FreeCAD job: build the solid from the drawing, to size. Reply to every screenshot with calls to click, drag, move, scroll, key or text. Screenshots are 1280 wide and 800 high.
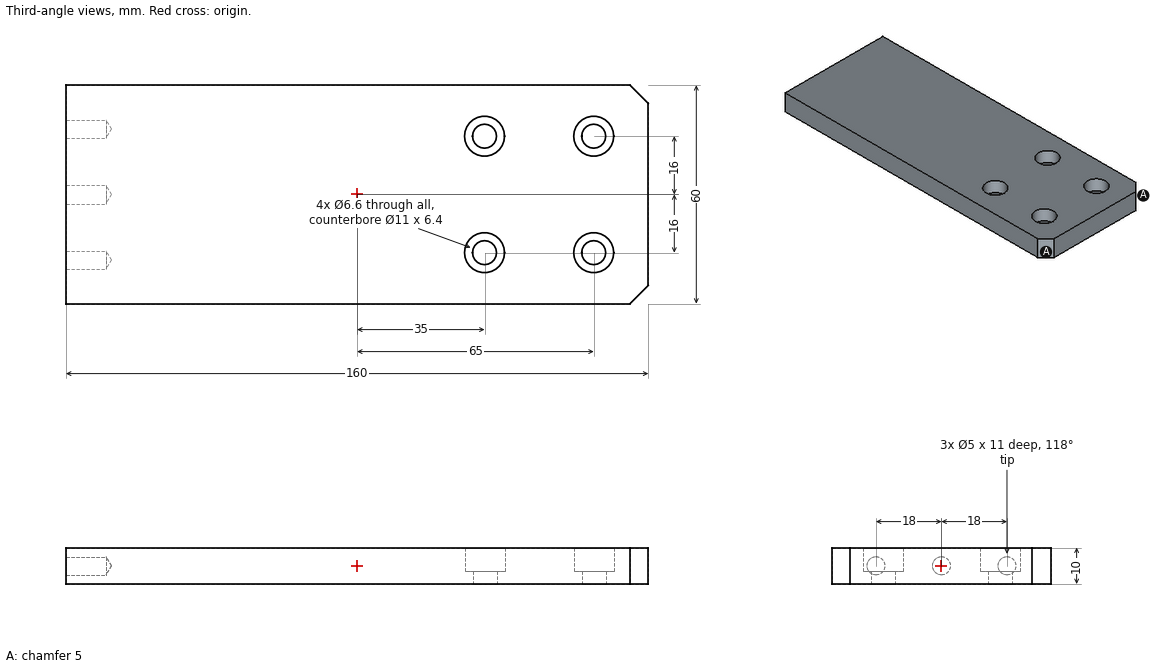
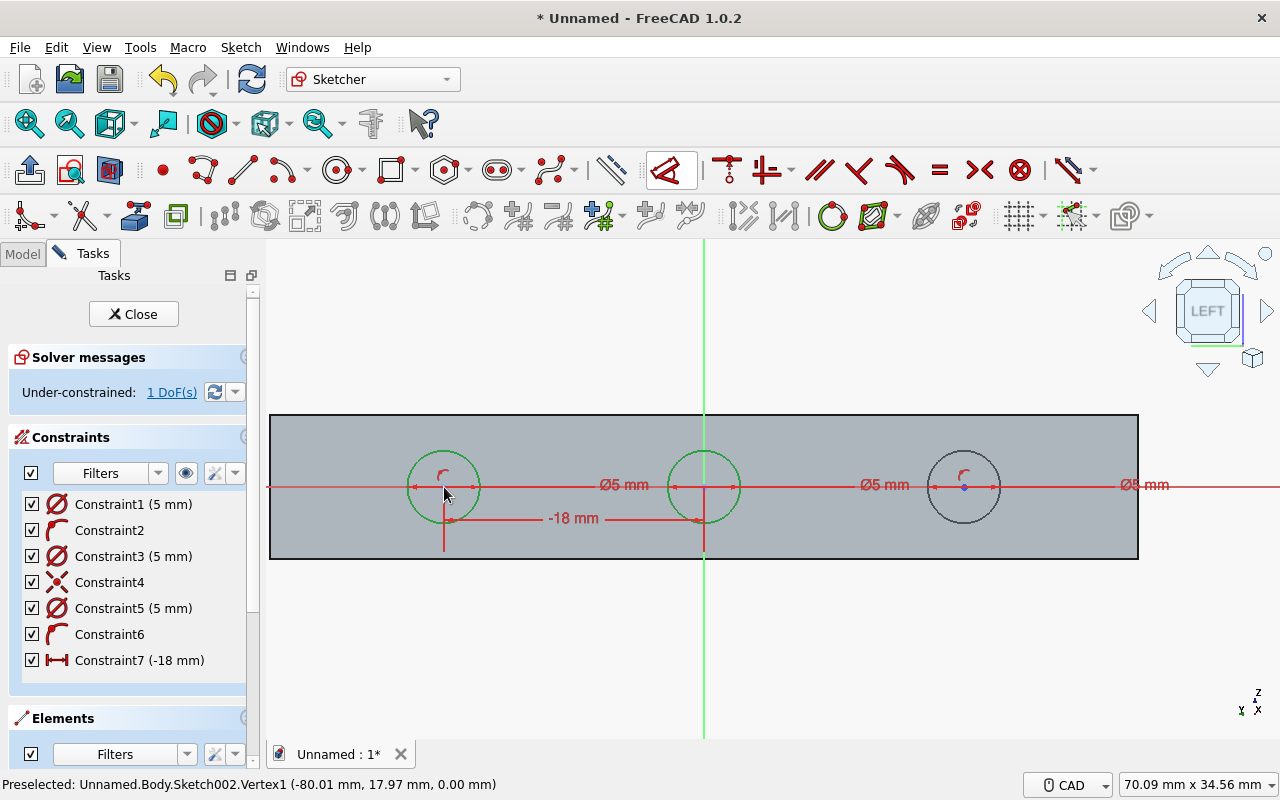
click(964, 487)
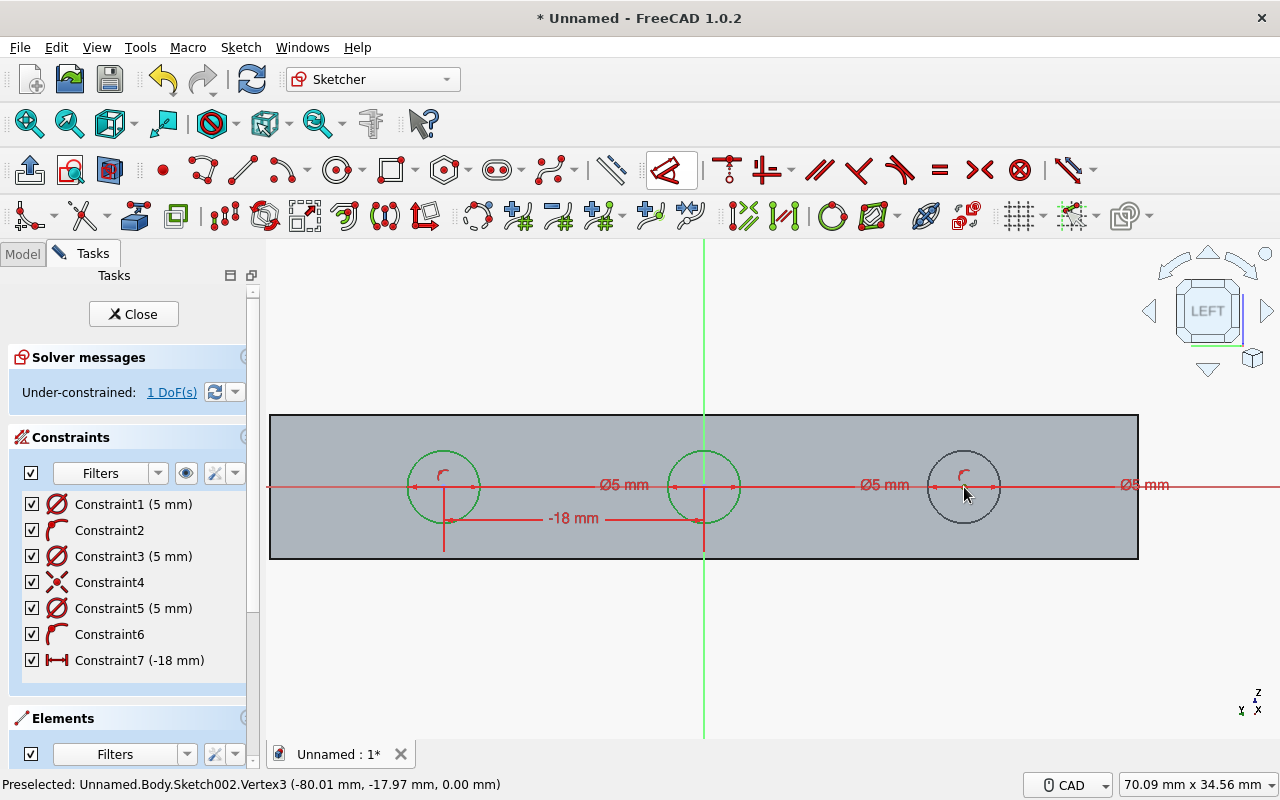
key(l)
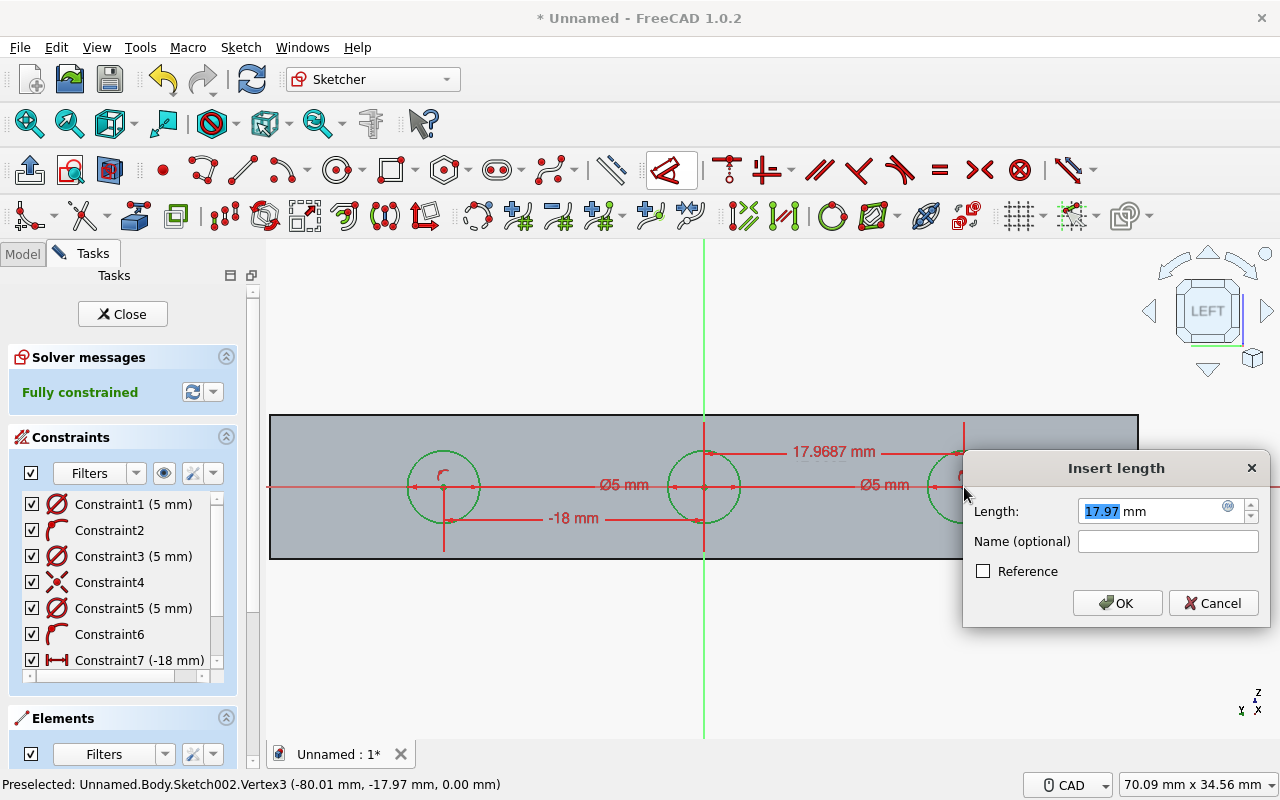
text(18)
key(Return)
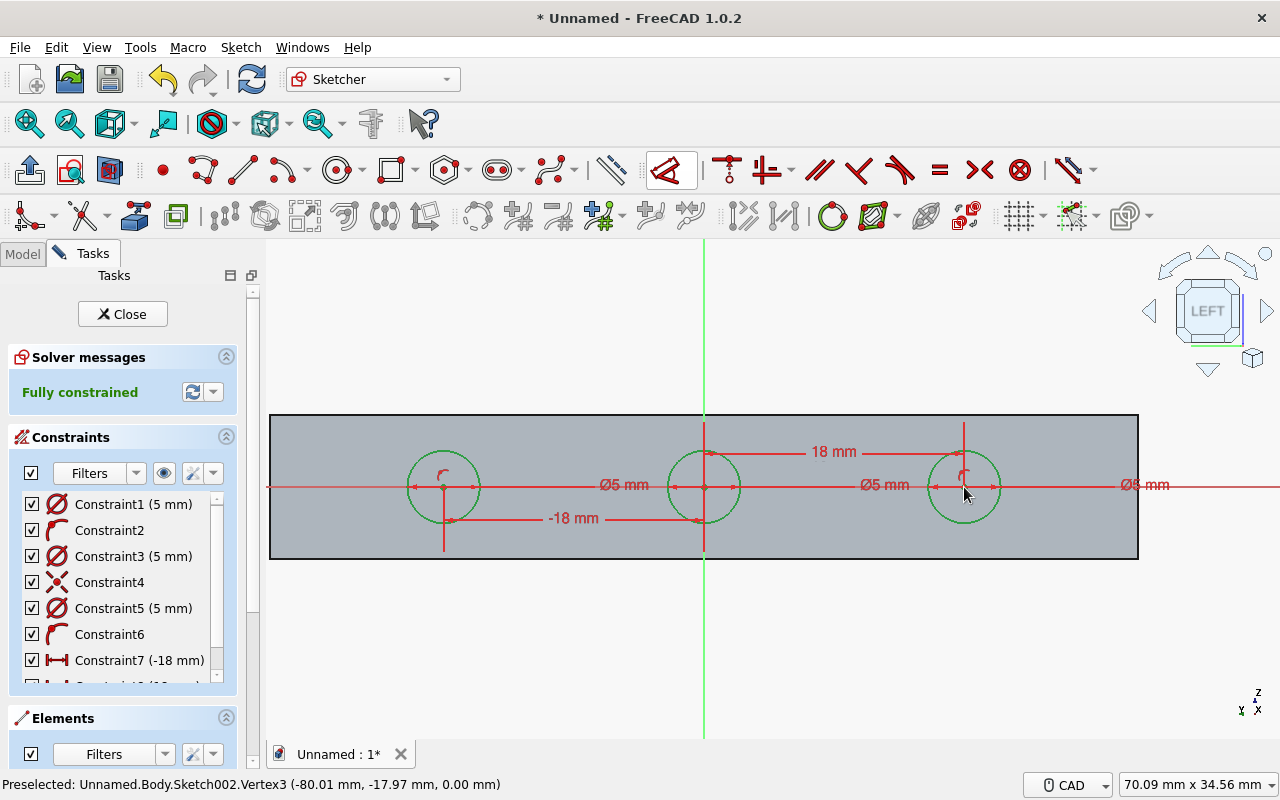
click(123, 314)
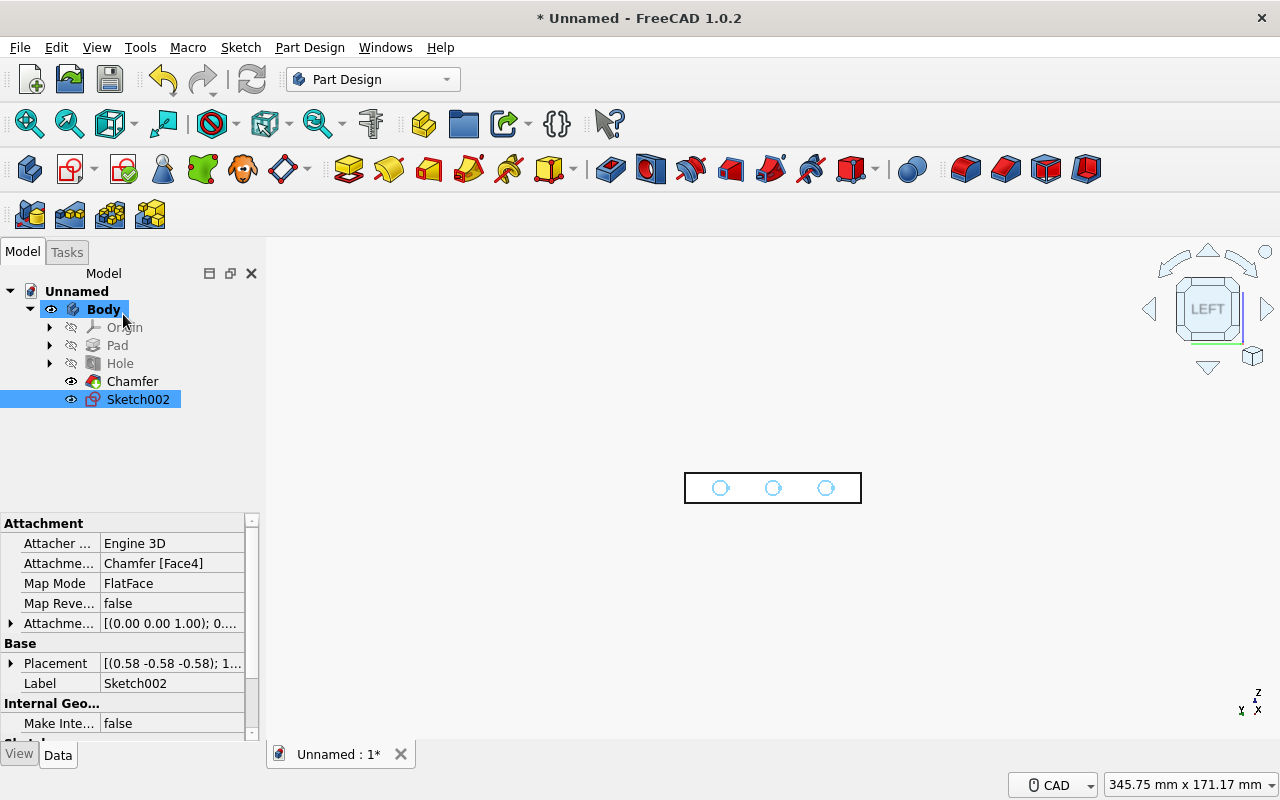
click(652, 170)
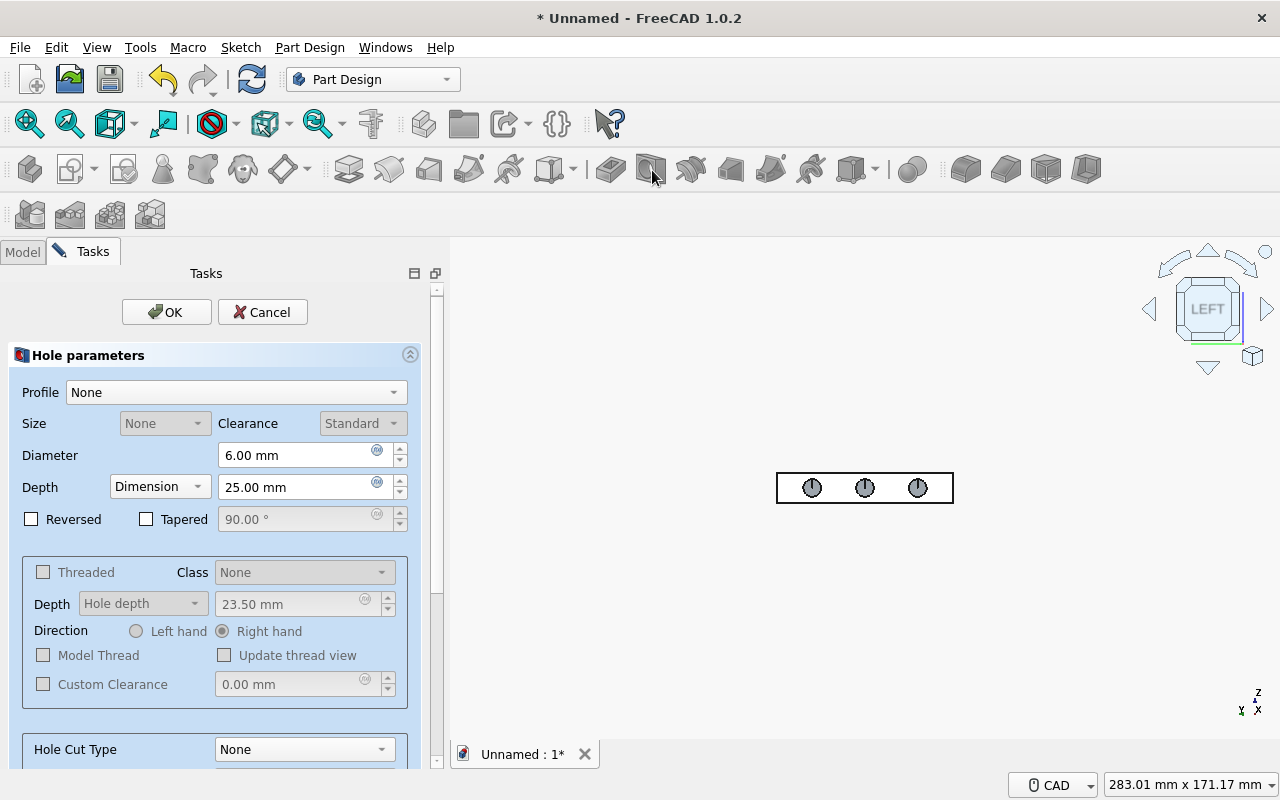
triple_click(305, 455)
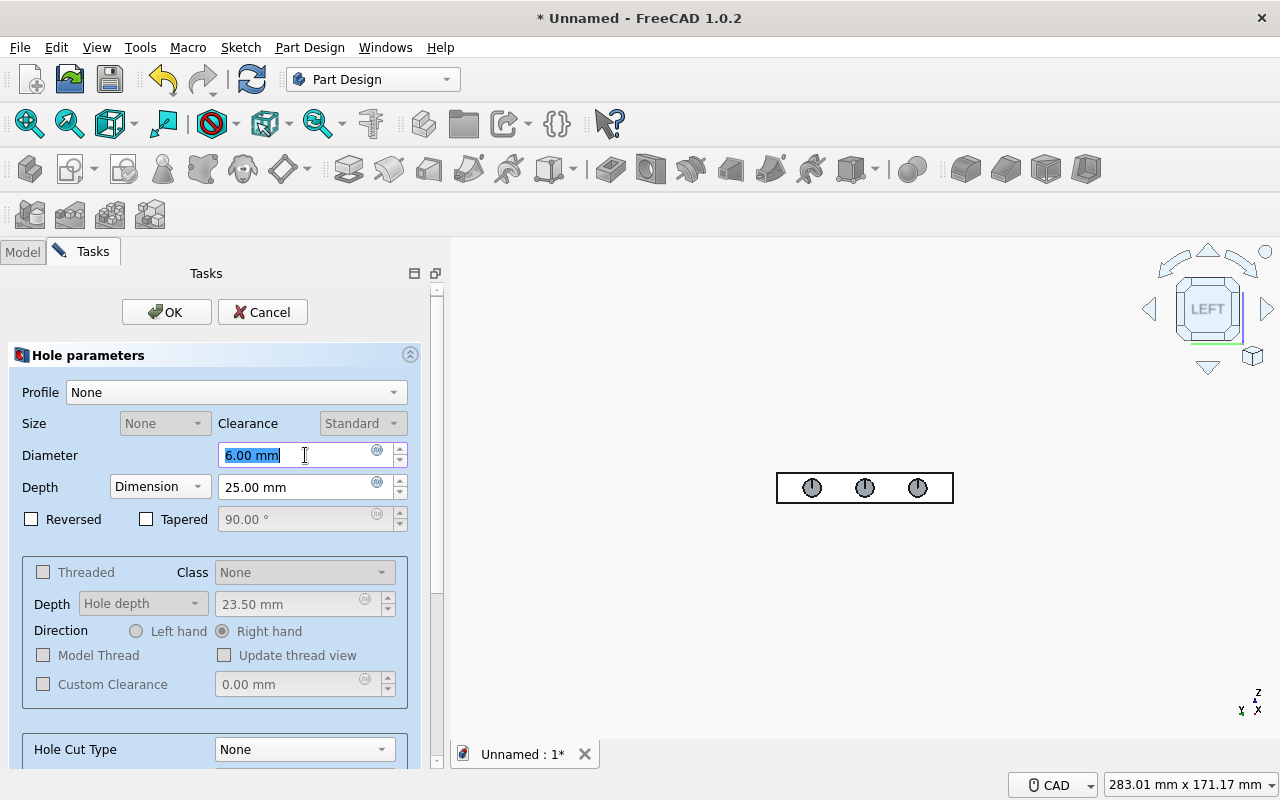
text(5)
key(Tab)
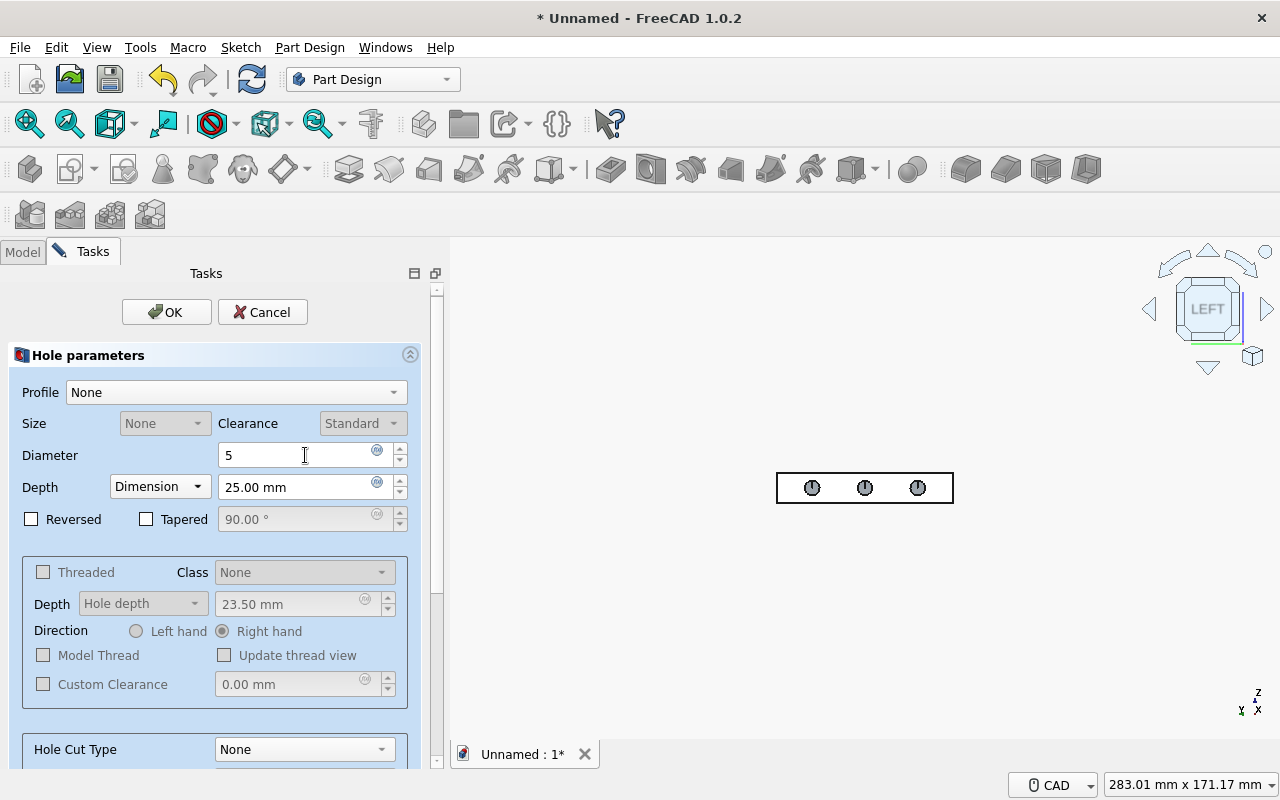
triple_click(305, 487)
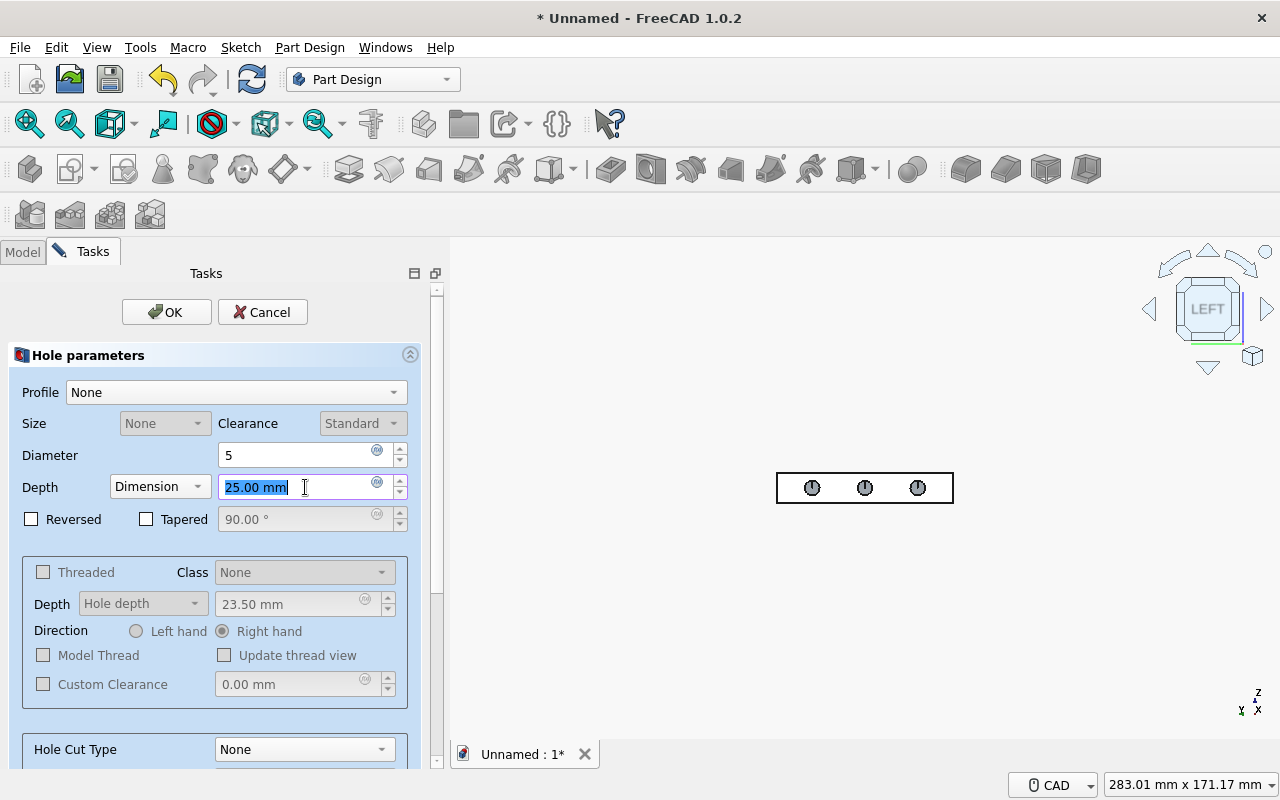
text(11)
key(Tab)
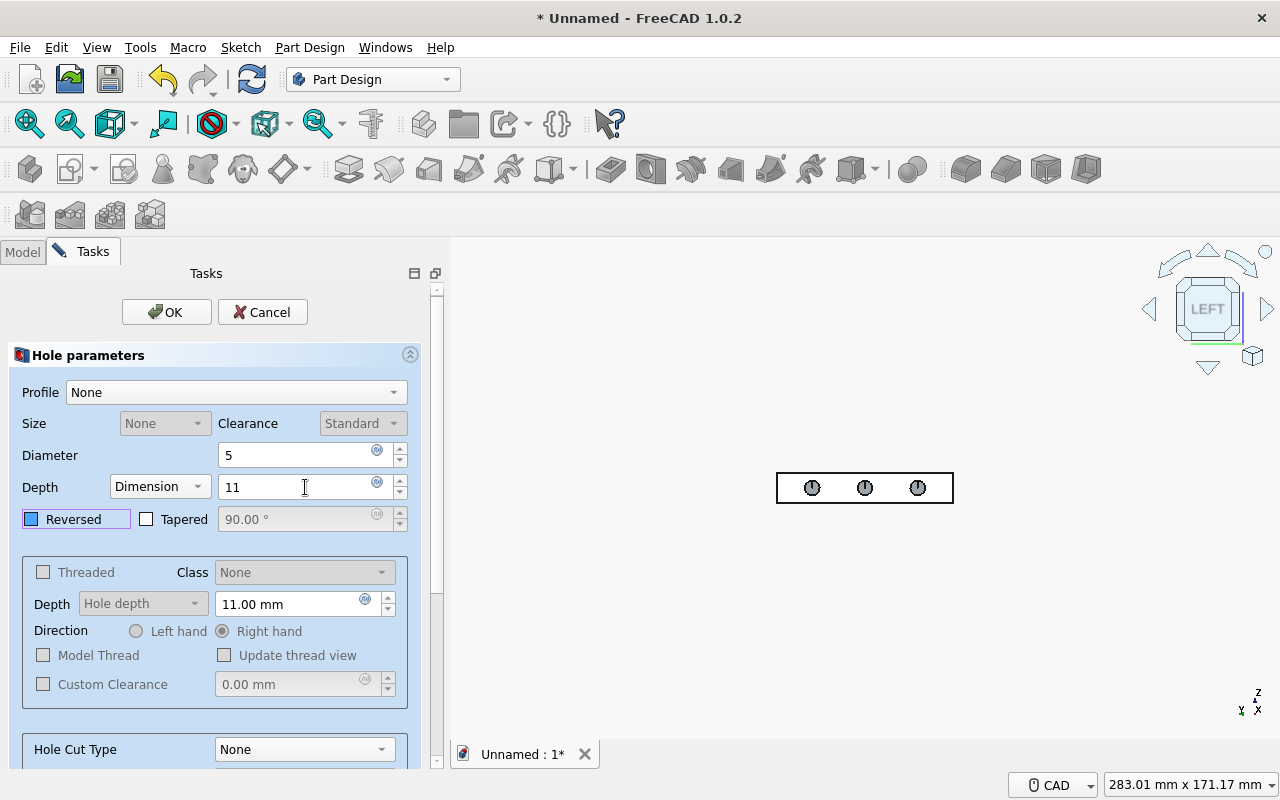
click(167, 312)